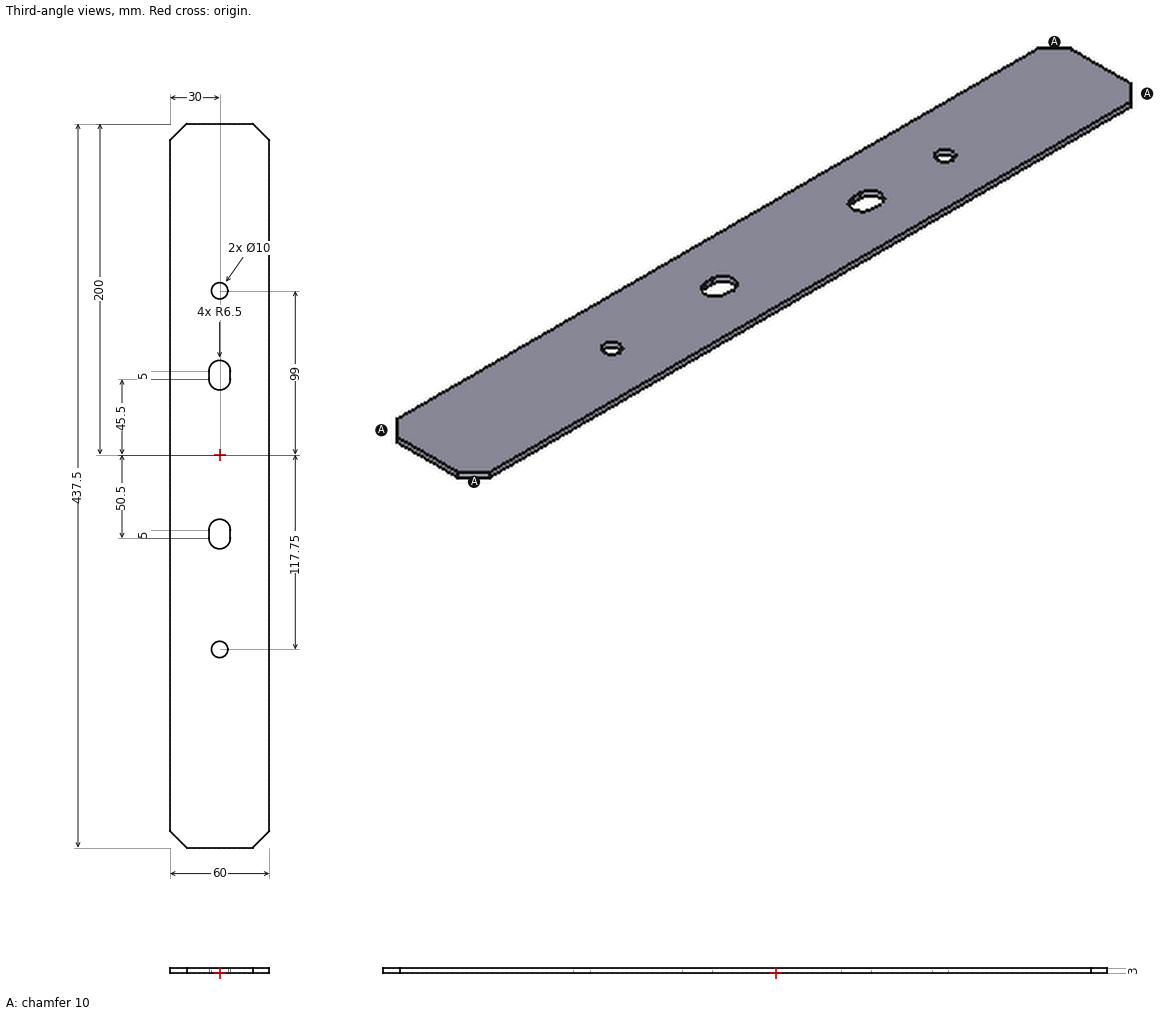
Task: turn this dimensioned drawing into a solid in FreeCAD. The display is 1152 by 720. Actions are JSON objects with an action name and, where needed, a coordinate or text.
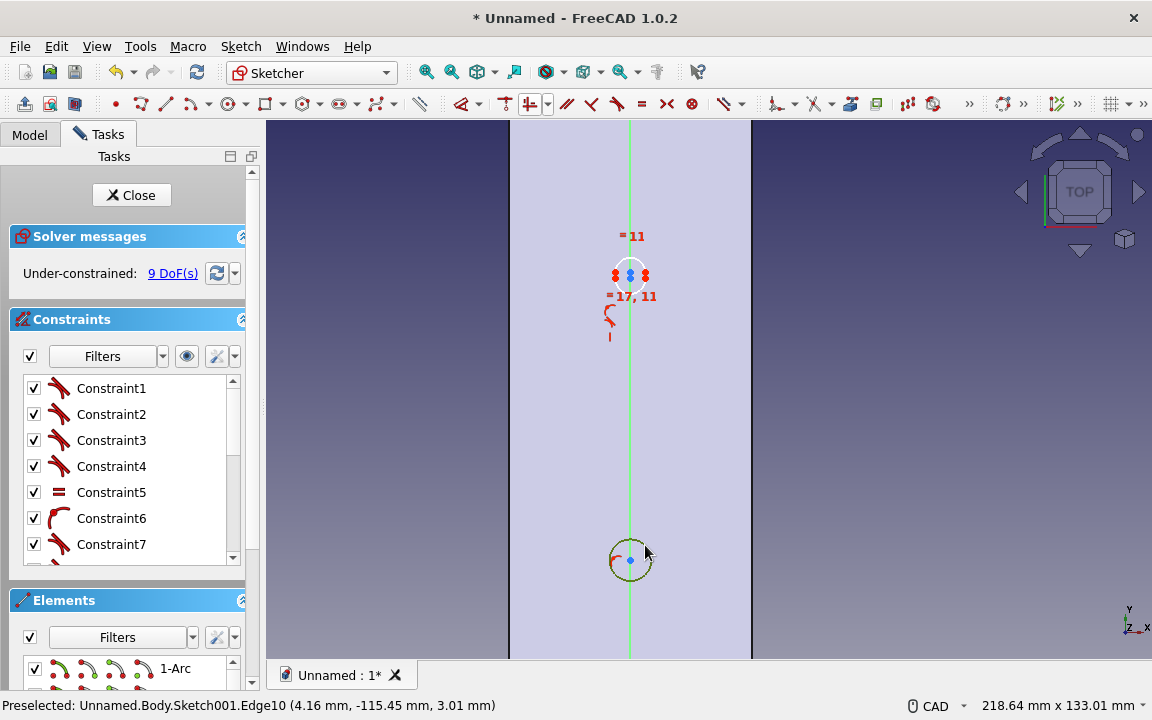
{"action": "key", "text": "e"}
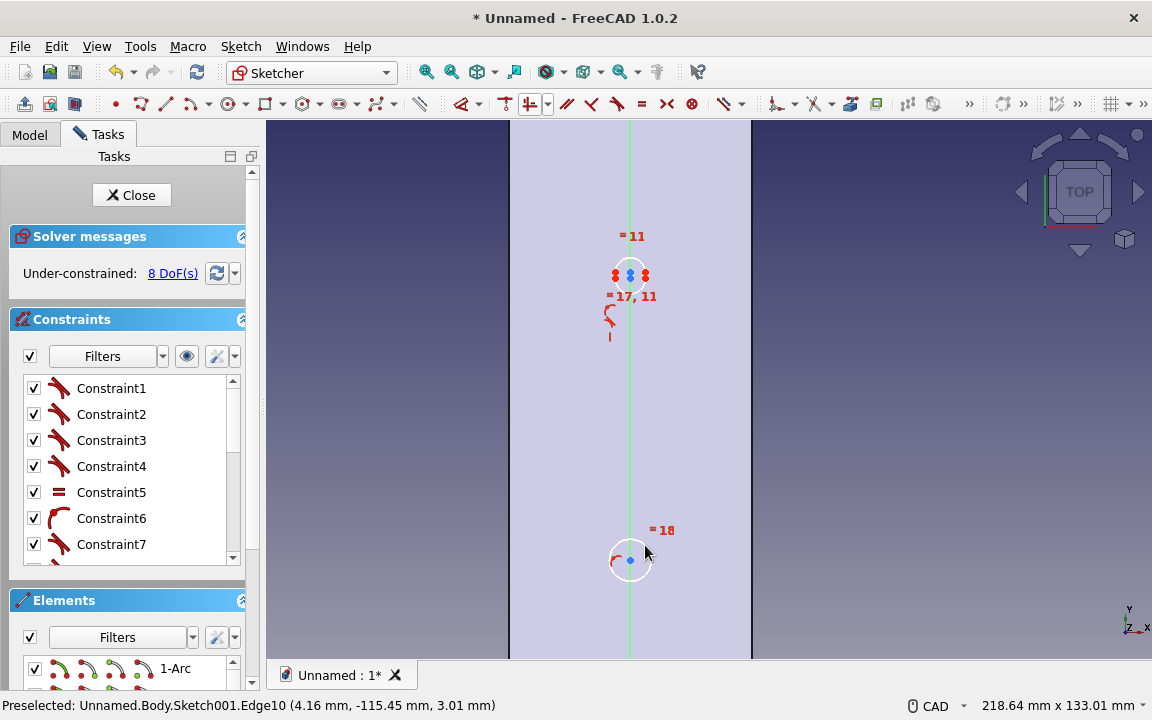
{"action": "key", "text": "d"}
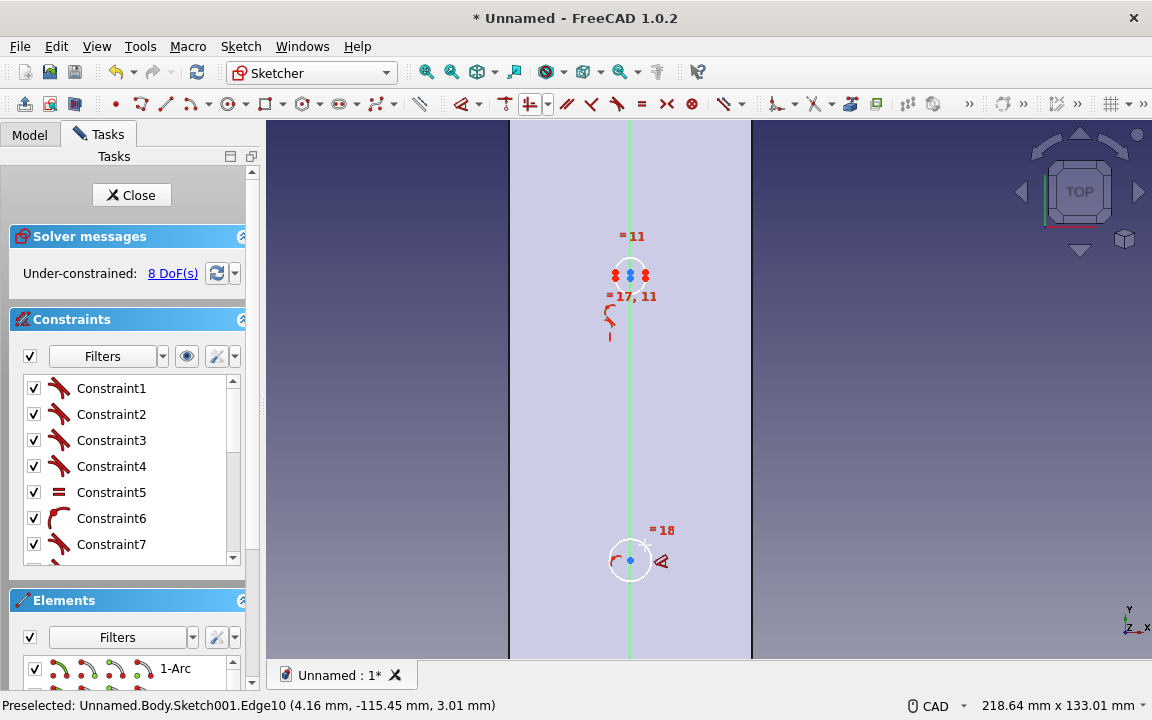
{"action": "scroll", "coordinate": [646, 547], "scroll_direction": "down", "scroll_amount": 5}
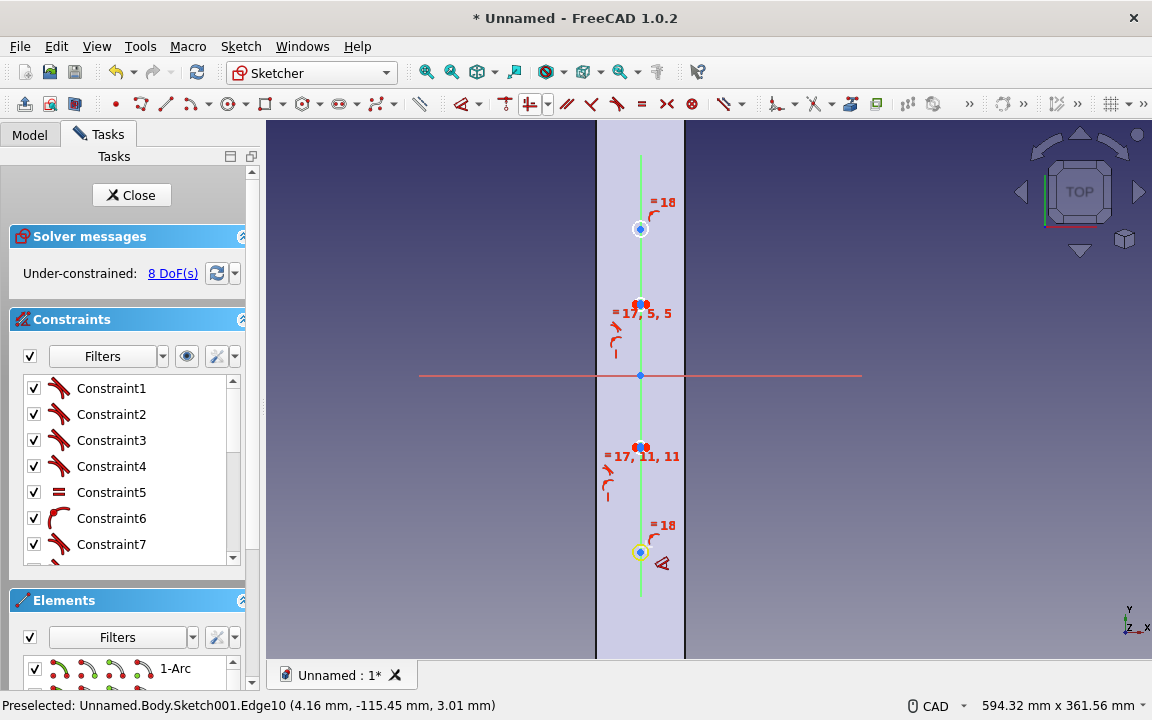
{"action": "scroll", "coordinate": [641, 311], "scroll_direction": "up", "scroll_amount": 8}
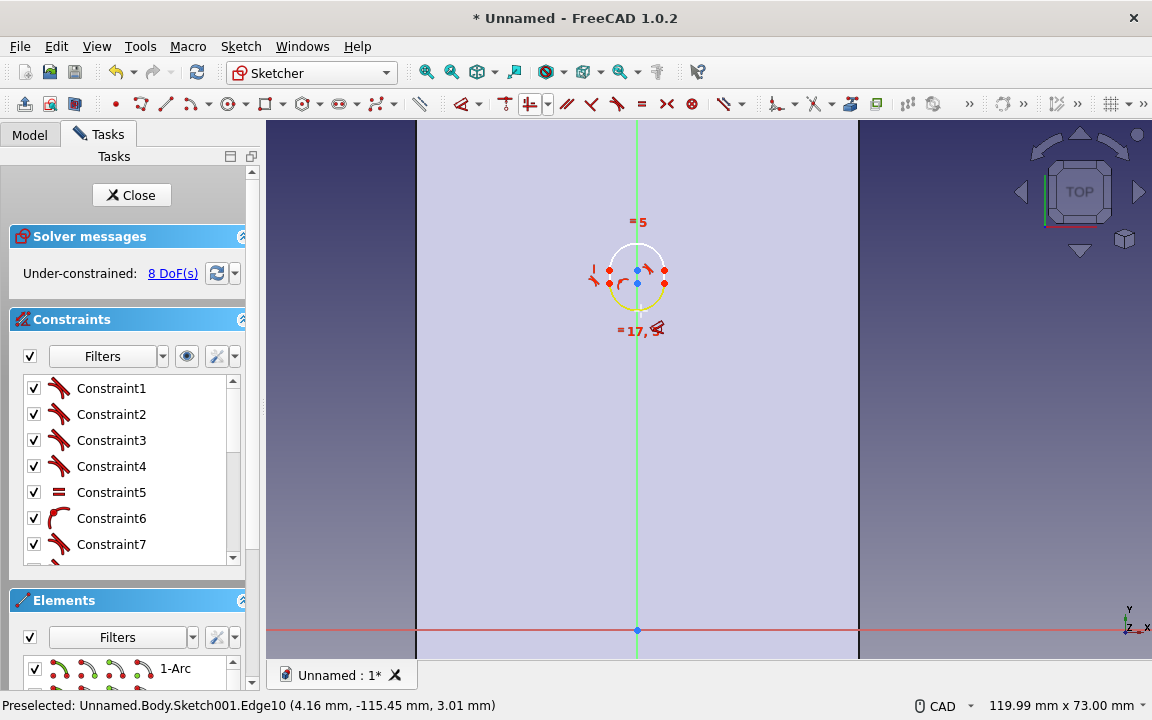
{"action": "left_click", "coordinate": [637, 310]}
{"action": "left_click", "coordinate": [609, 335]}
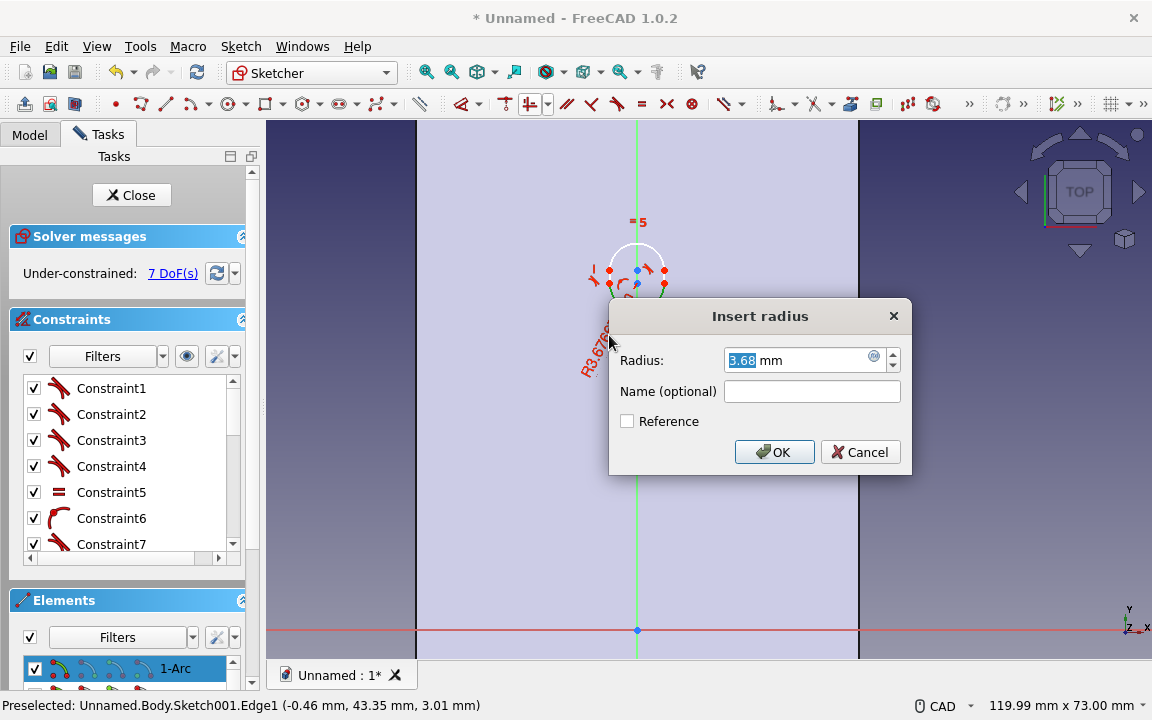
{"action": "type", "text": "6.5"}
{"action": "key", "text": "Return"}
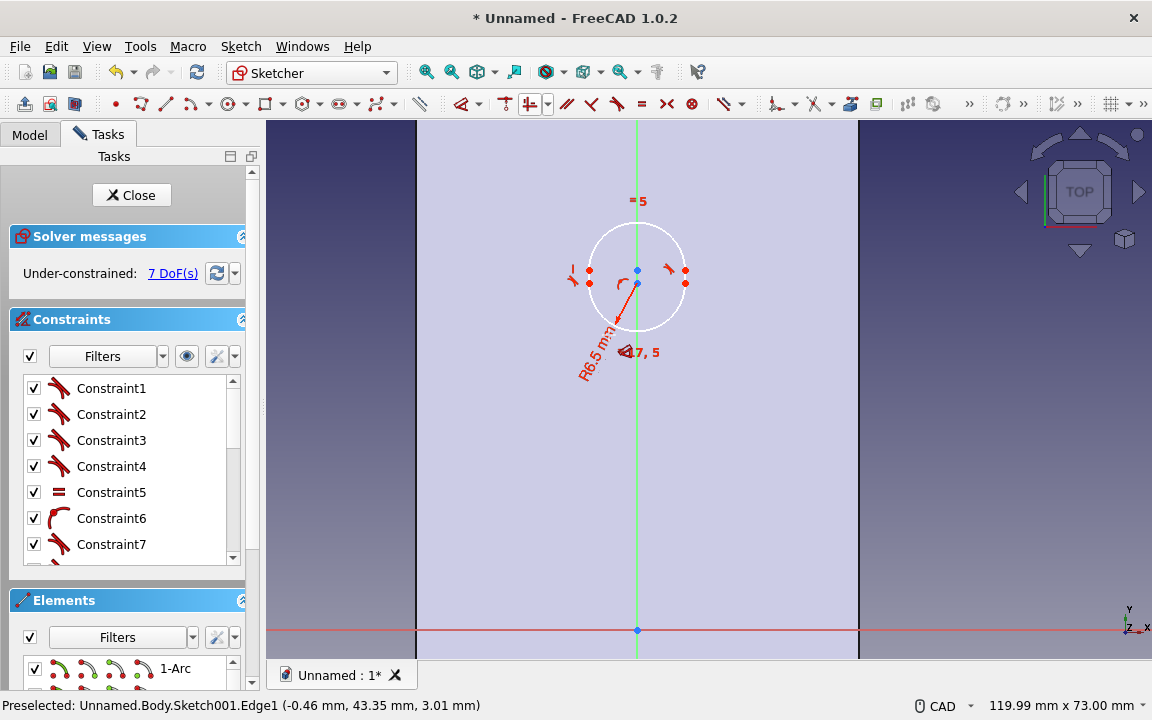
{"action": "scroll", "coordinate": [641, 311], "scroll_direction": "down", "scroll_amount": 8}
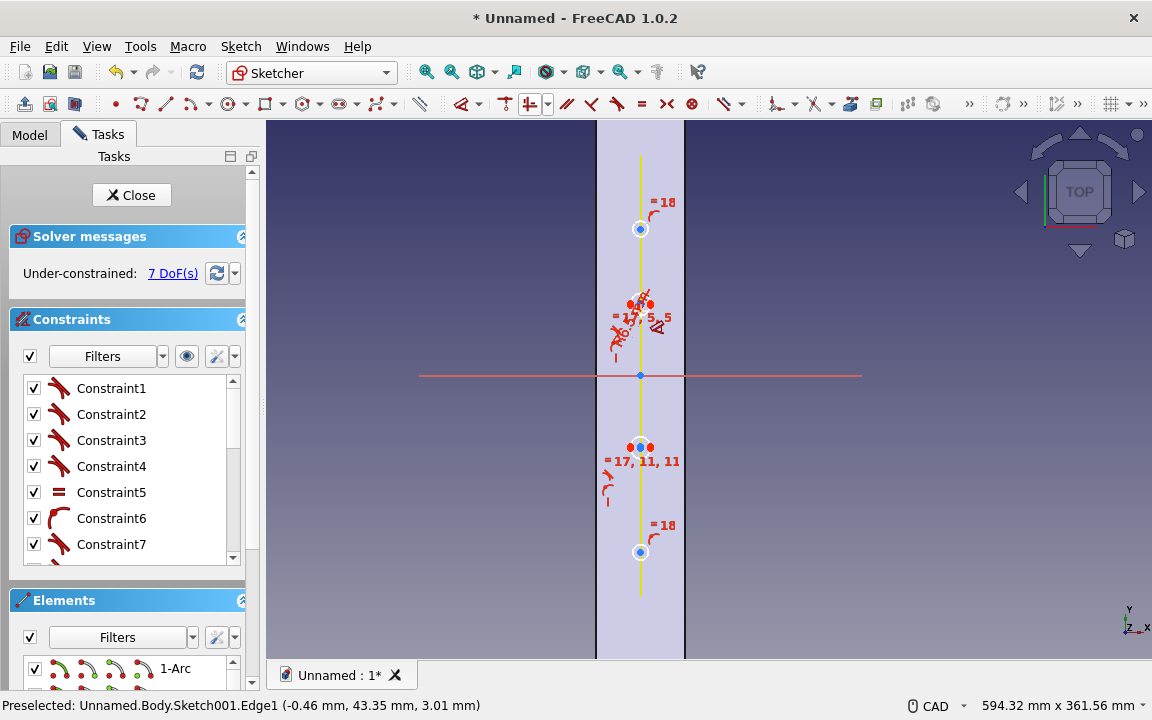
{"action": "scroll", "coordinate": [646, 224], "scroll_direction": "up", "scroll_amount": 5}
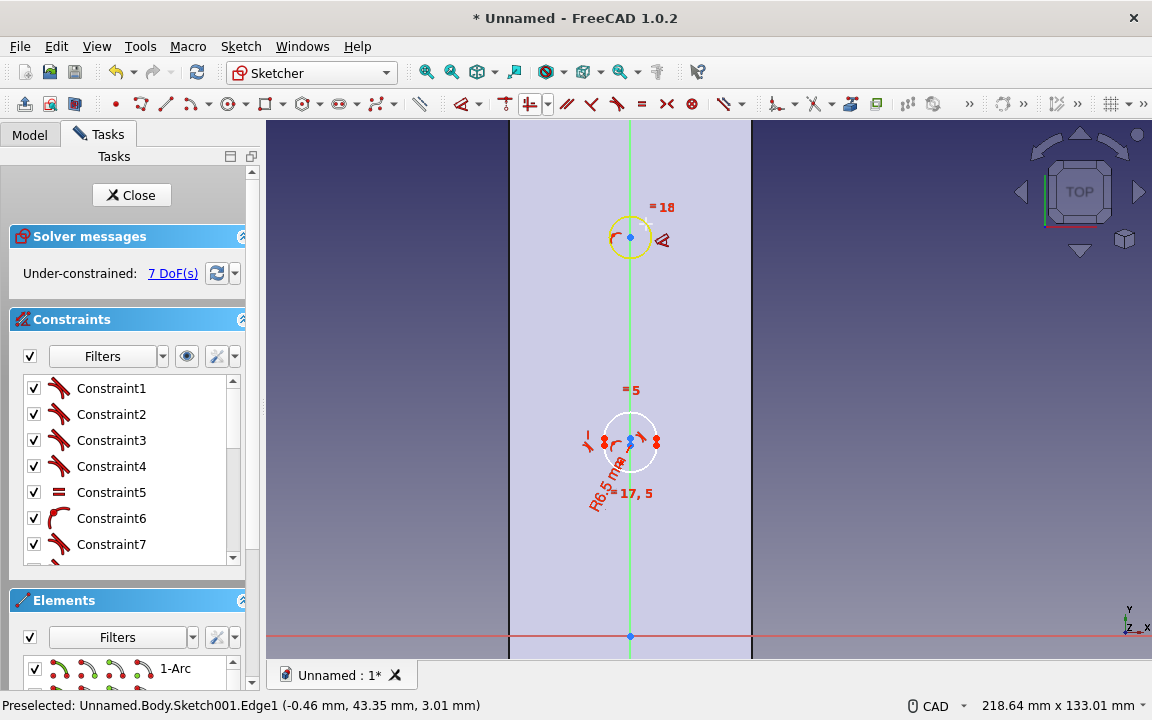
{"action": "left_click", "coordinate": [645, 223]}
{"action": "left_click", "coordinate": [668, 200]}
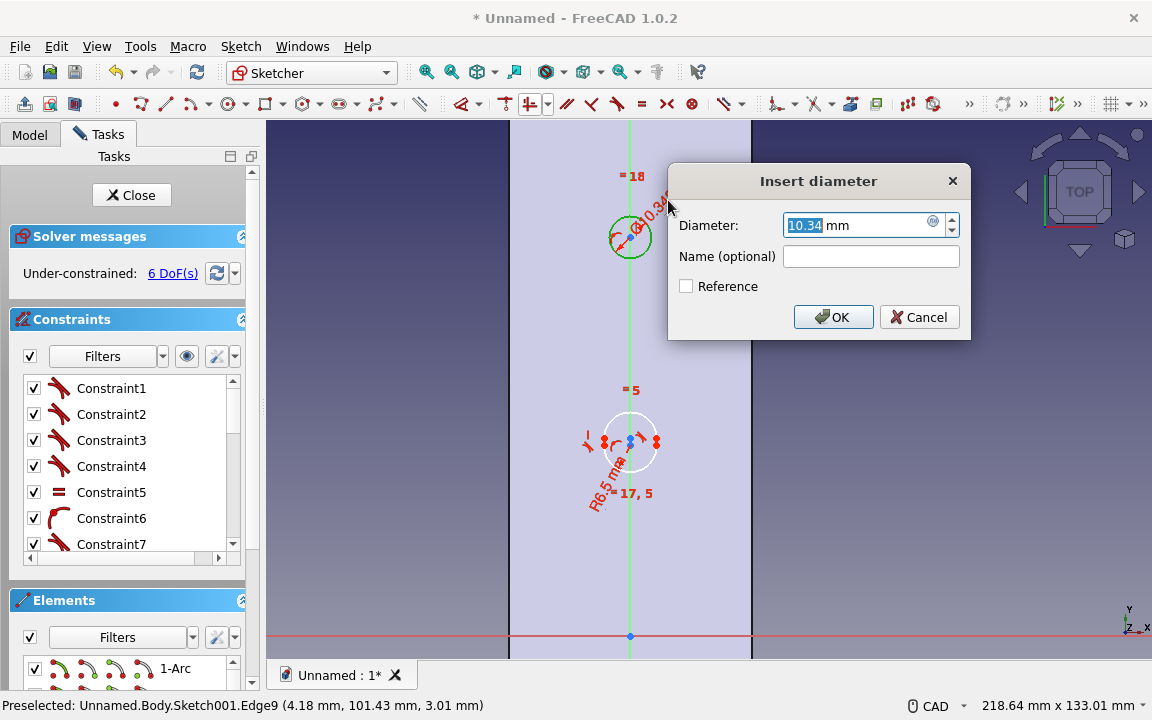
{"action": "type", "text": "10"}
{"action": "key", "text": "Return"}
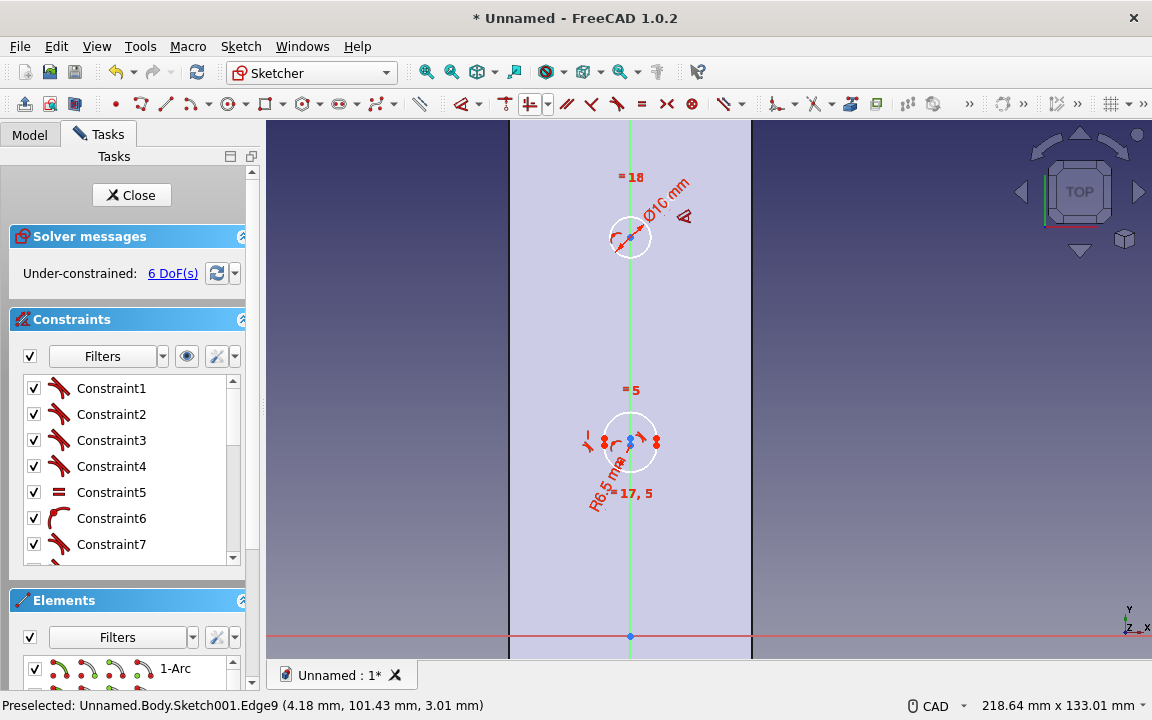
{"action": "scroll", "coordinate": [604, 442], "scroll_direction": "up", "scroll_amount": 7}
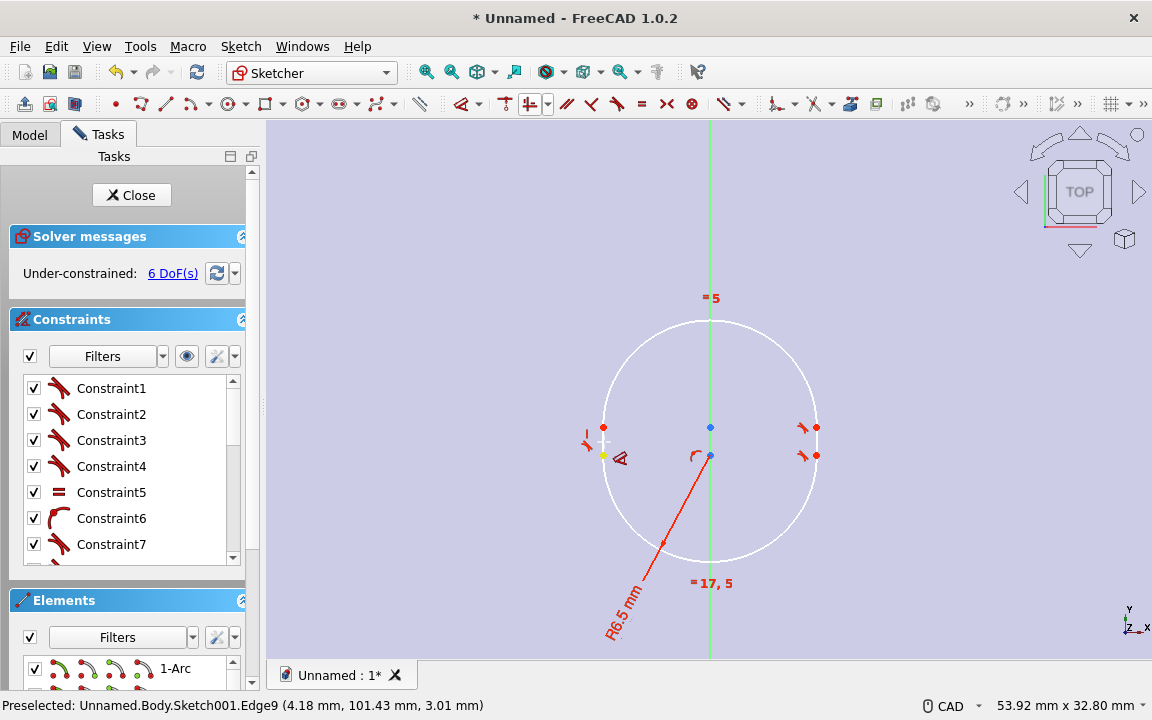
{"action": "left_click", "coordinate": [603, 441]}
{"action": "left_click", "coordinate": [569, 441]}